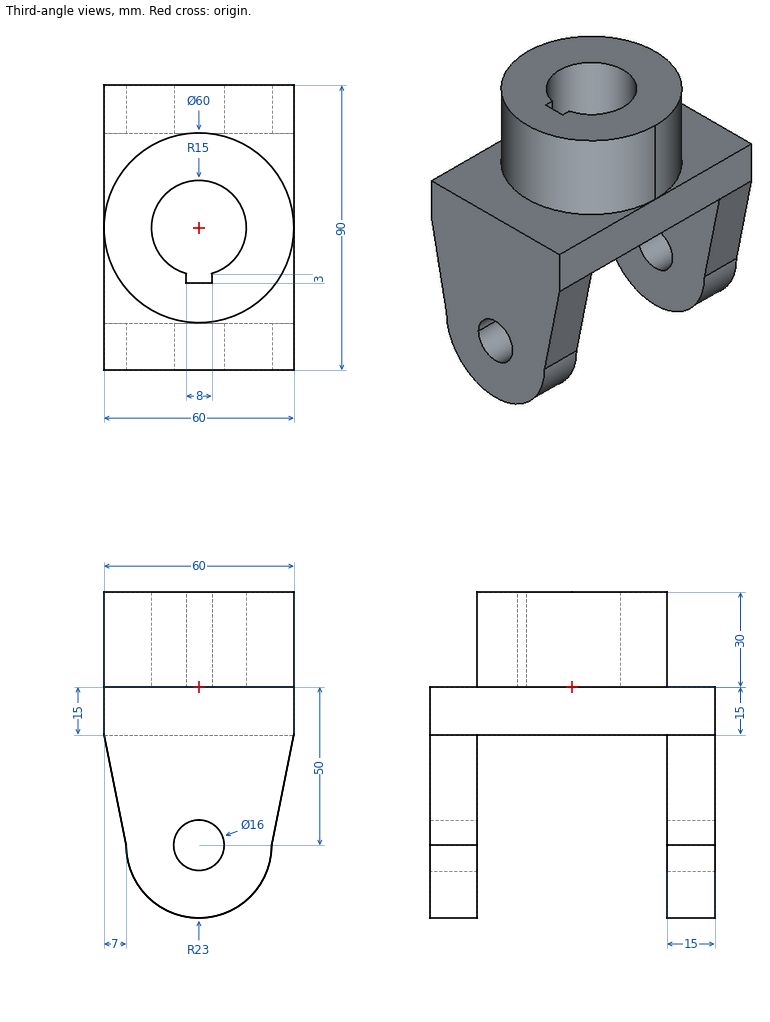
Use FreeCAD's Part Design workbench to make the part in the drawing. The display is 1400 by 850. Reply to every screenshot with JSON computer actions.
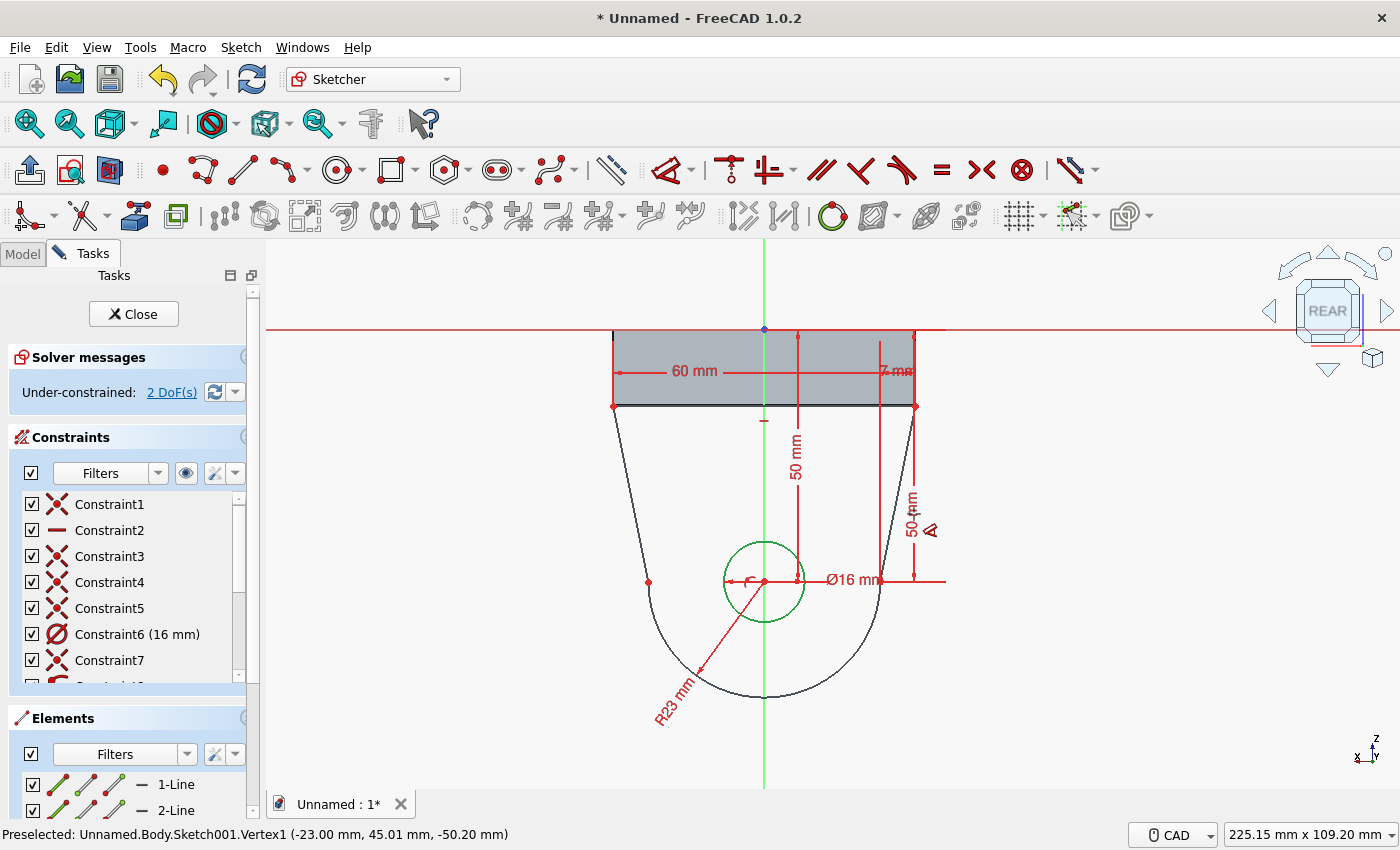
{"action": "left_click", "coordinate": [915, 406]}
{"action": "left_click", "coordinate": [949, 351]}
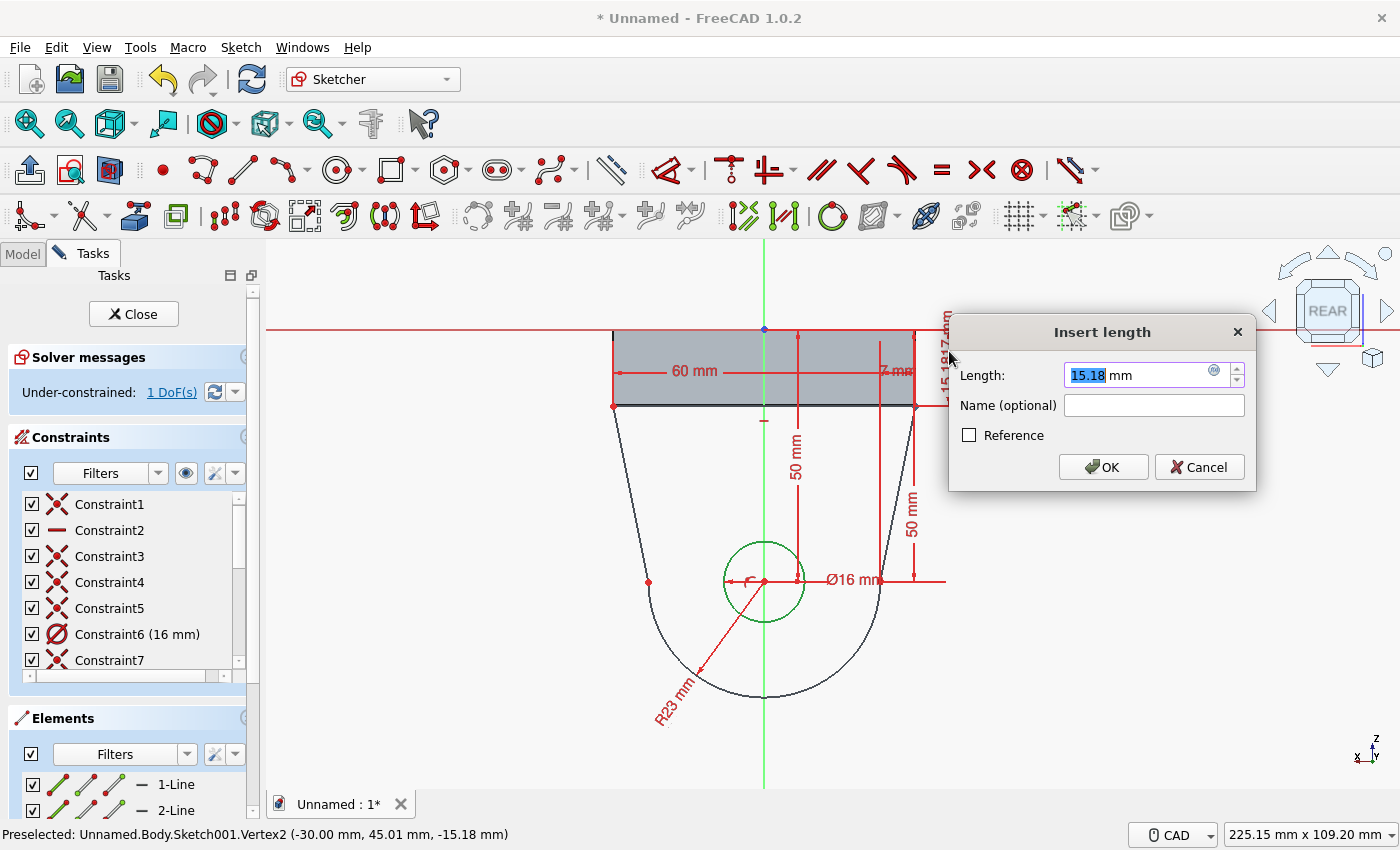
{"action": "type", "text": "15"}
{"action": "key", "text": "Return"}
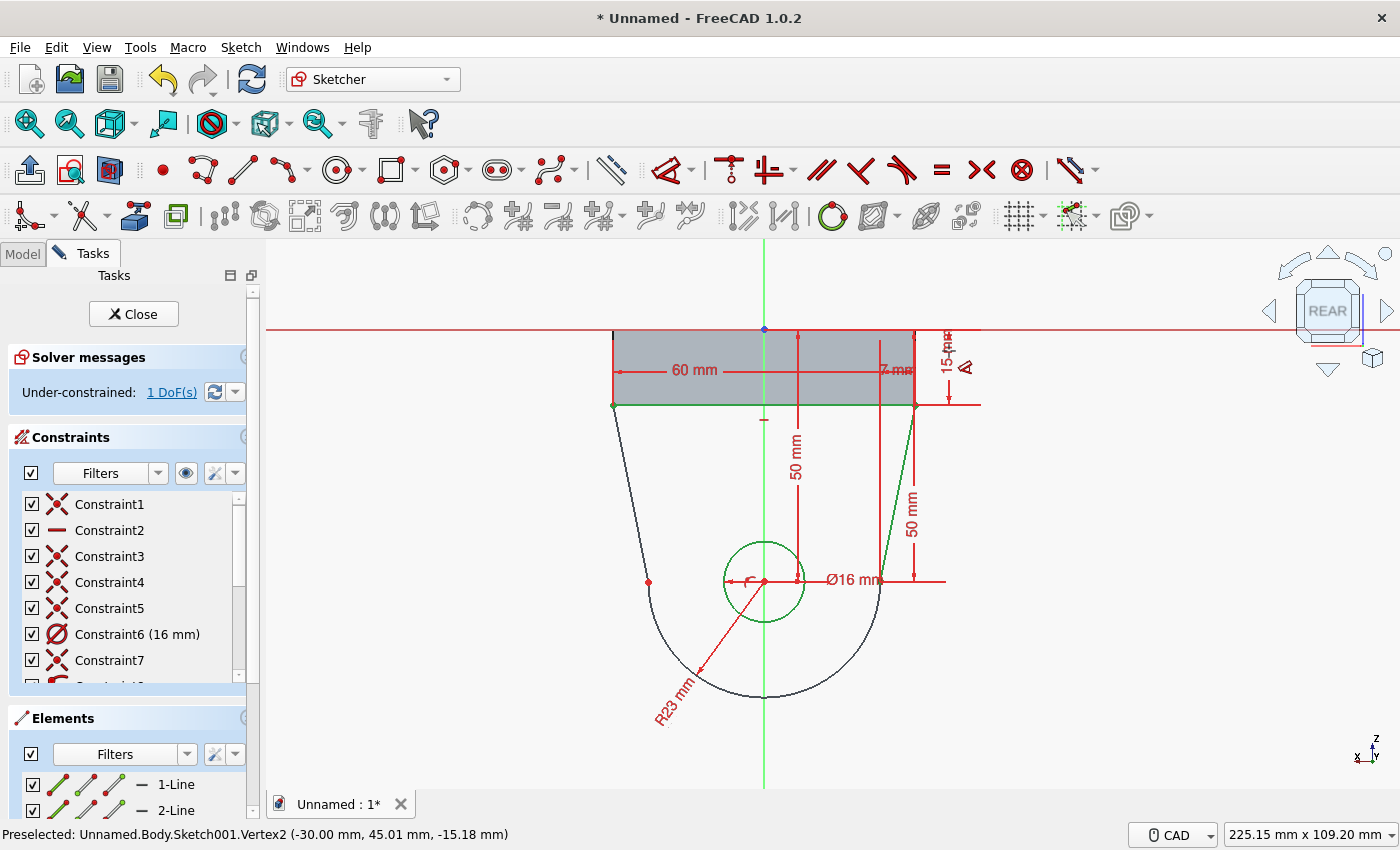
{"action": "left_click", "coordinate": [648, 583]}
{"action": "left_click", "coordinate": [614, 514]}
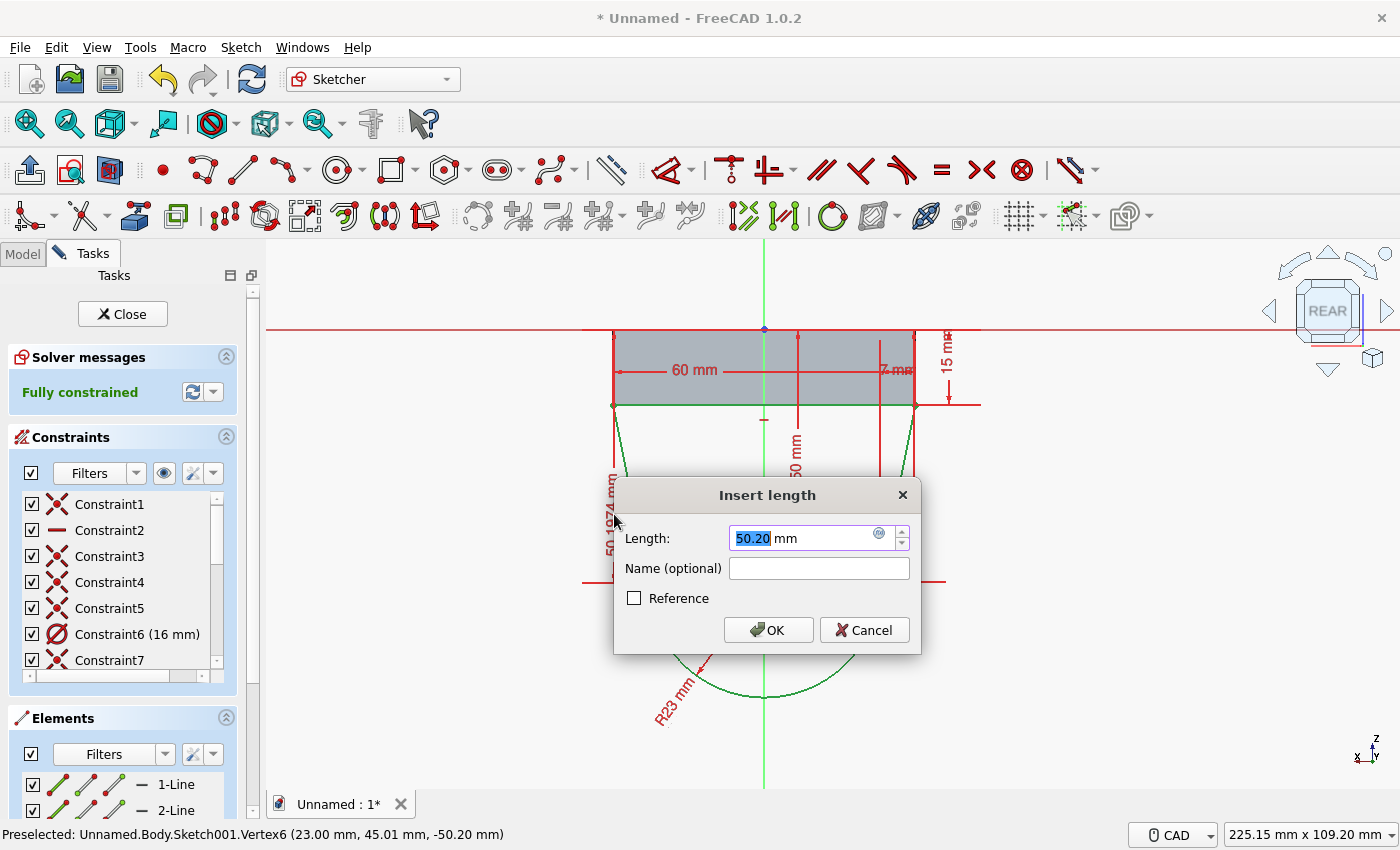
{"action": "type", "text": "50"}
{"action": "key", "text": "Return"}
{"action": "key", "text": "Escape"}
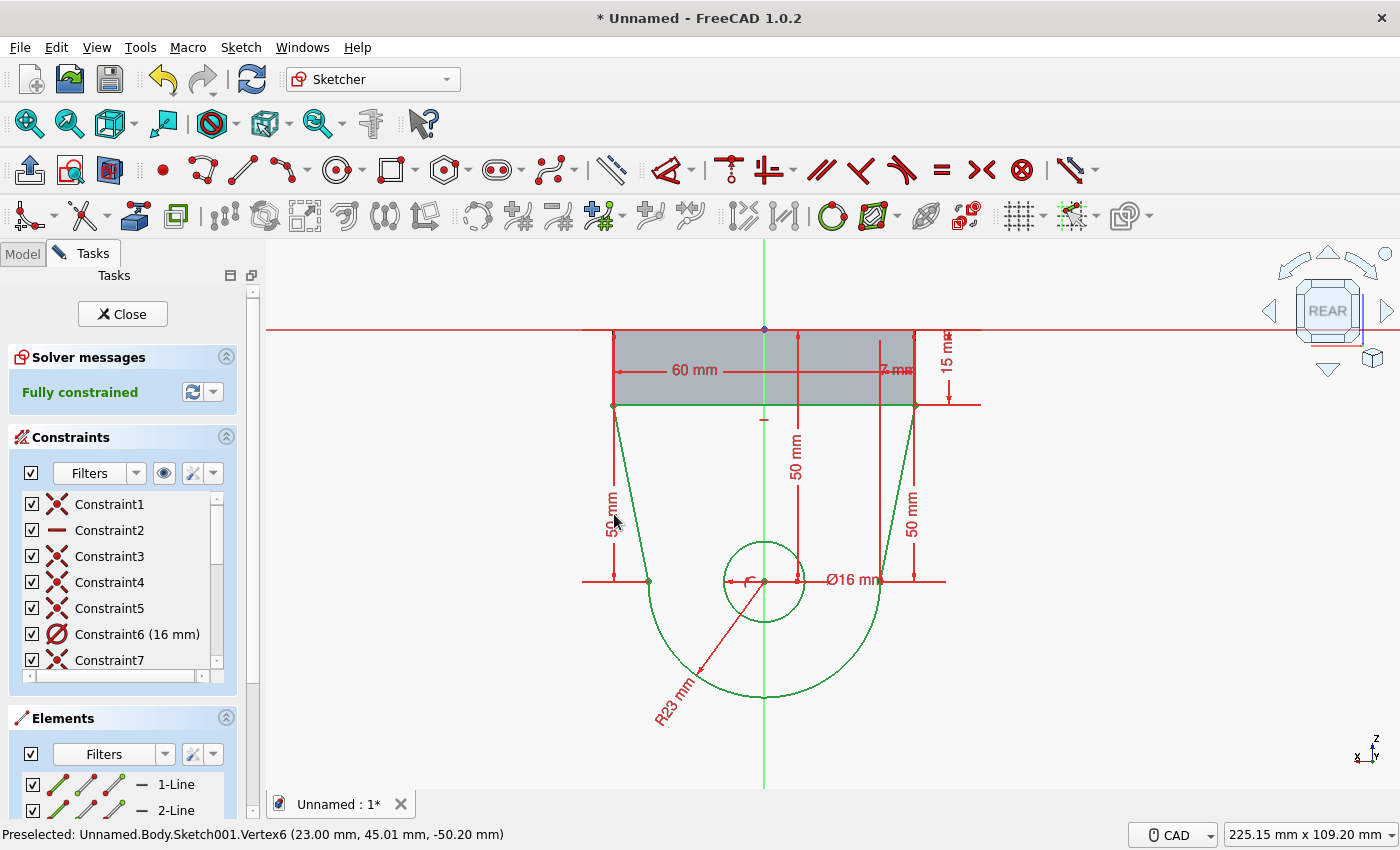
{"action": "left_click", "coordinate": [123, 314]}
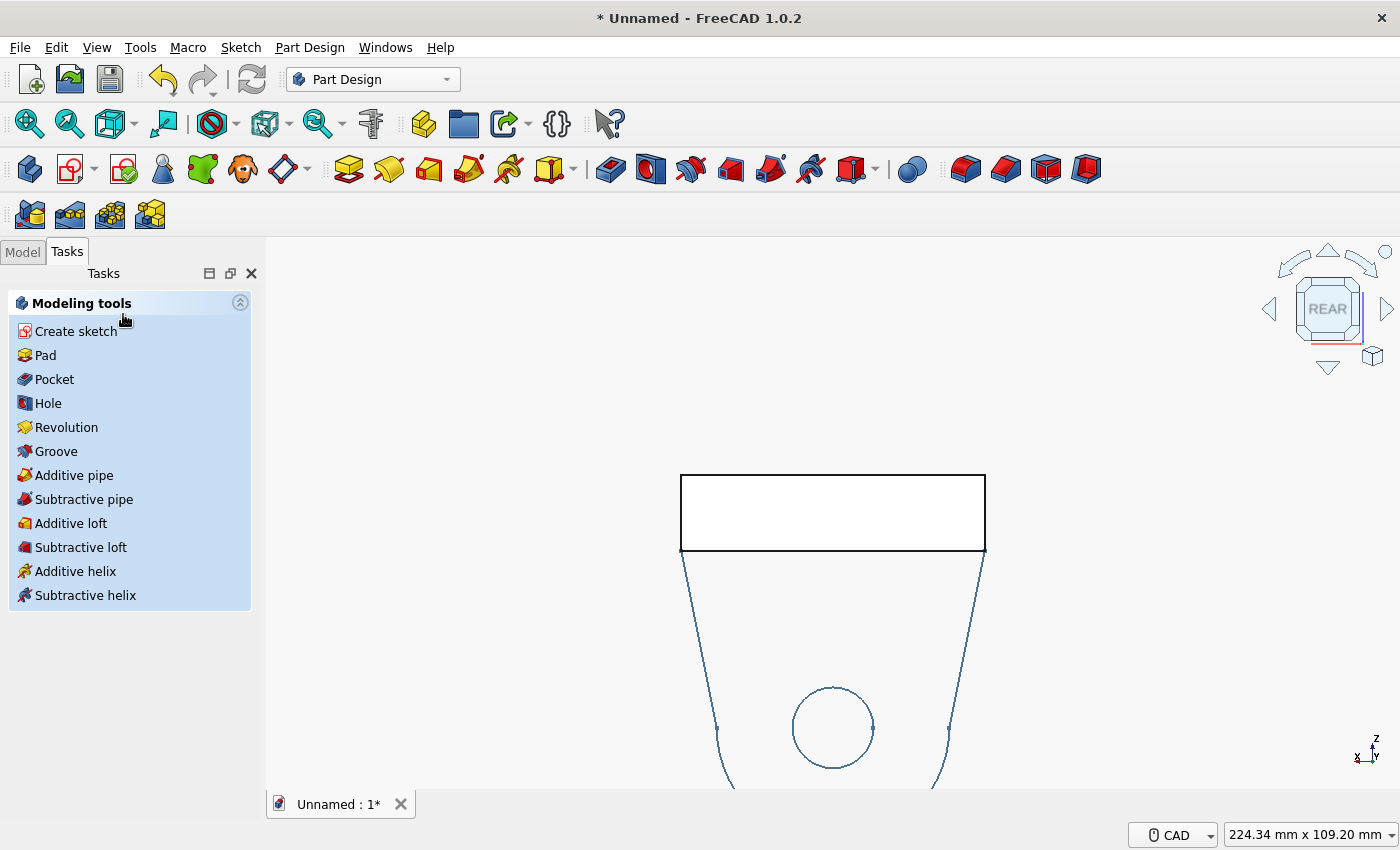
{"action": "left_click", "coordinate": [350, 170]}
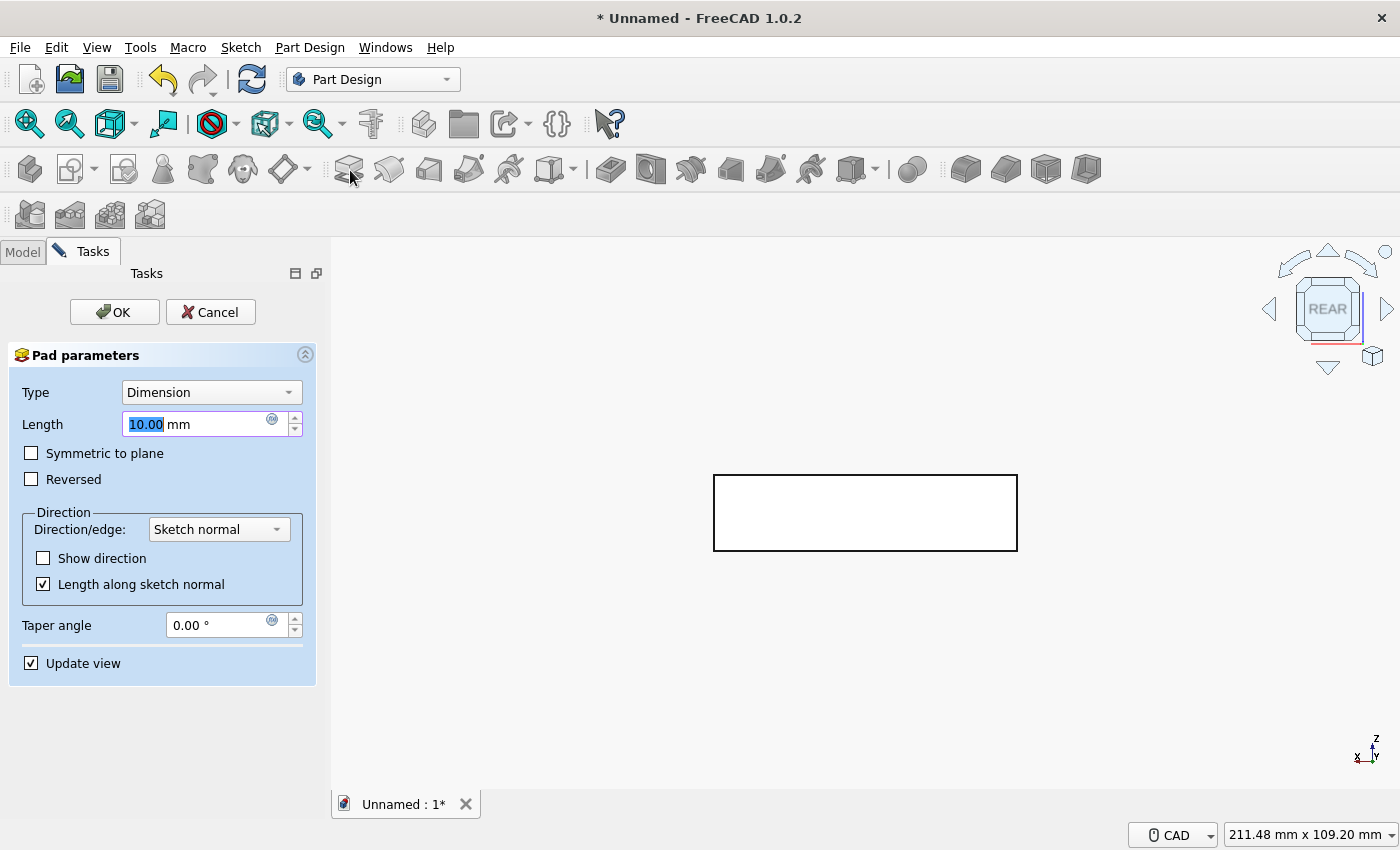
{"action": "type", "text": "15"}
{"action": "key", "text": "Tab"}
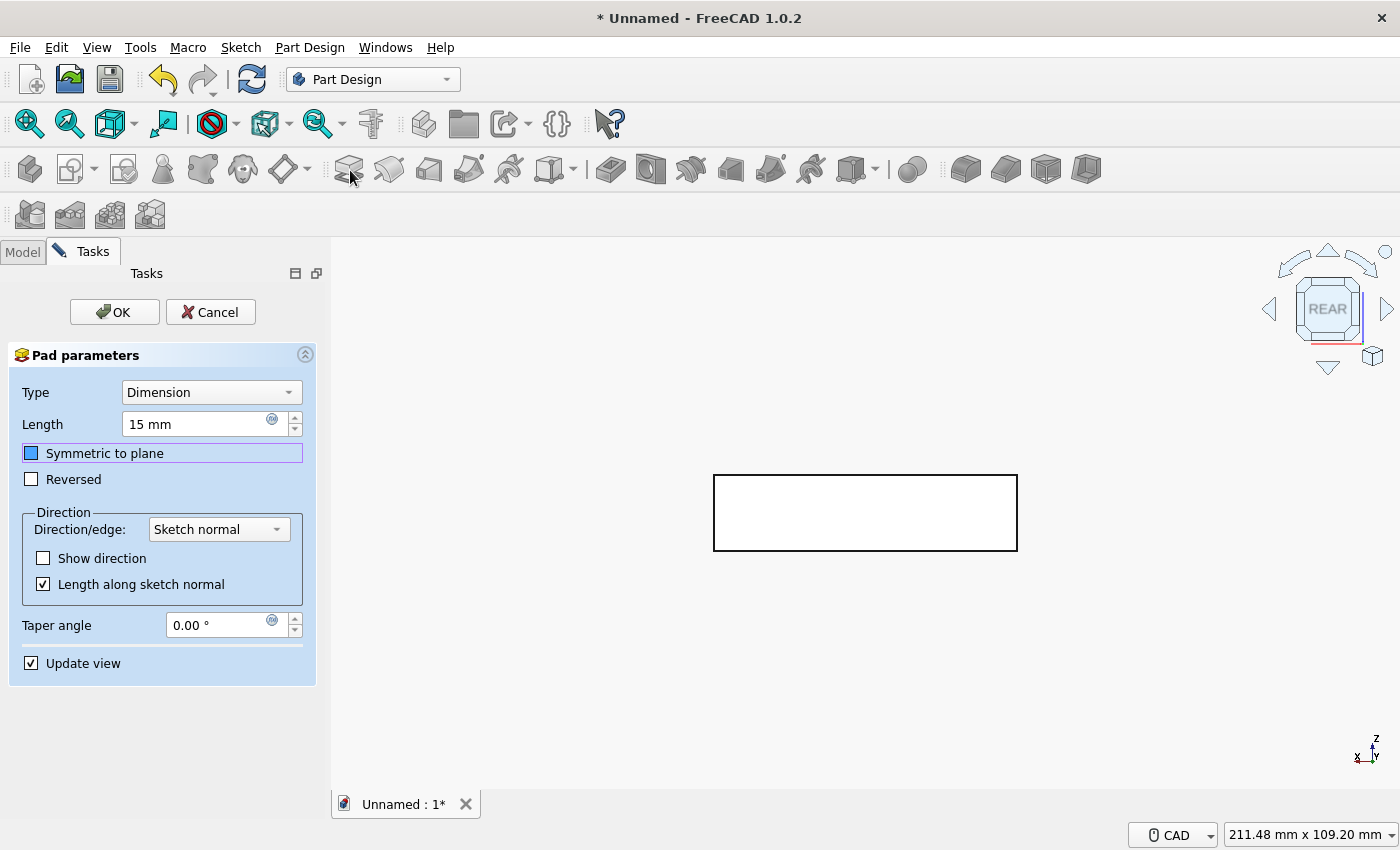
{"action": "left_click", "coordinate": [30, 479]}